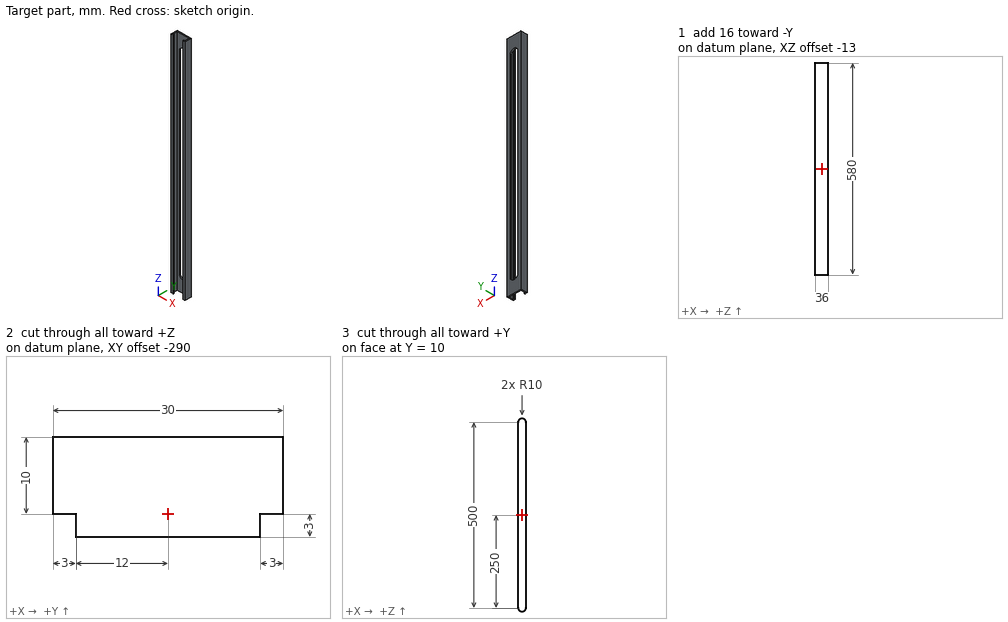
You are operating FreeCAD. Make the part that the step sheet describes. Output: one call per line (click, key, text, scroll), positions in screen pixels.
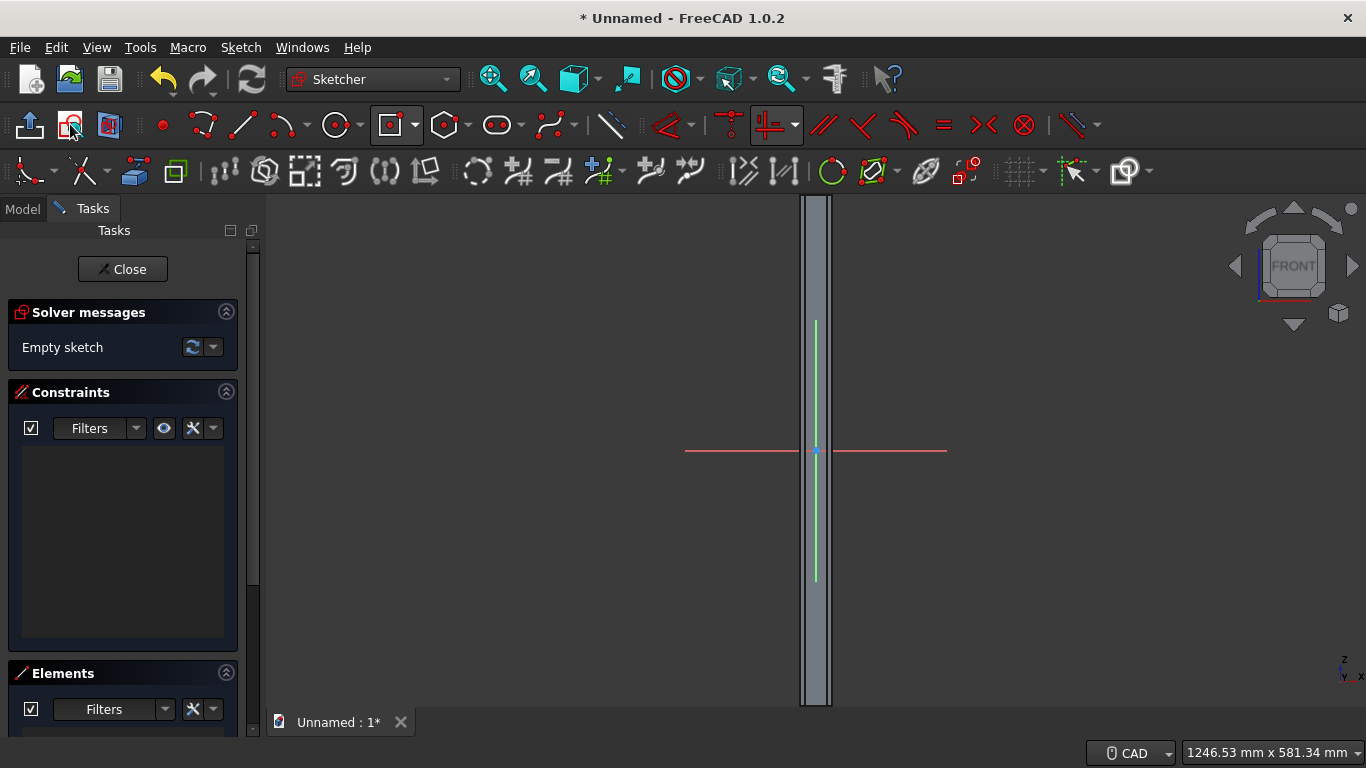
click(110, 126)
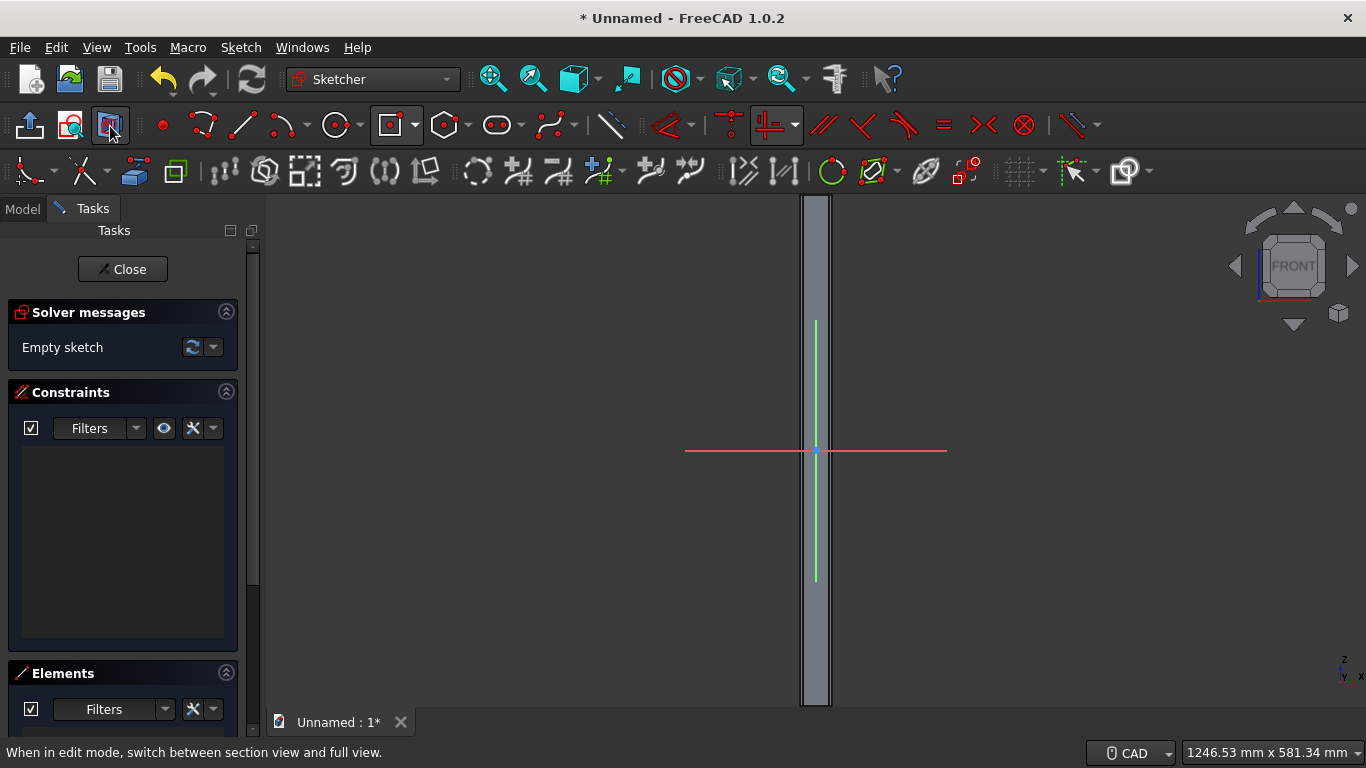
scroll(608, 450, down, 2)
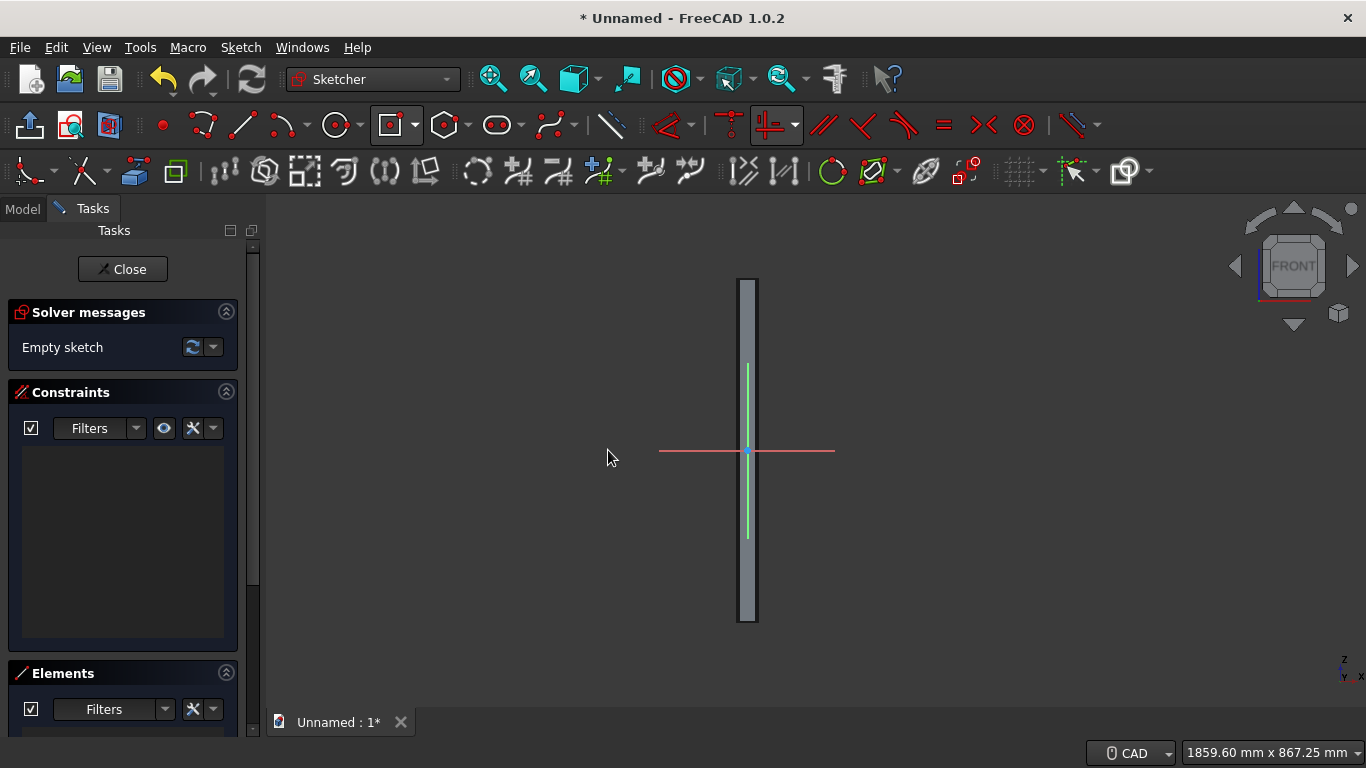
click(498, 126)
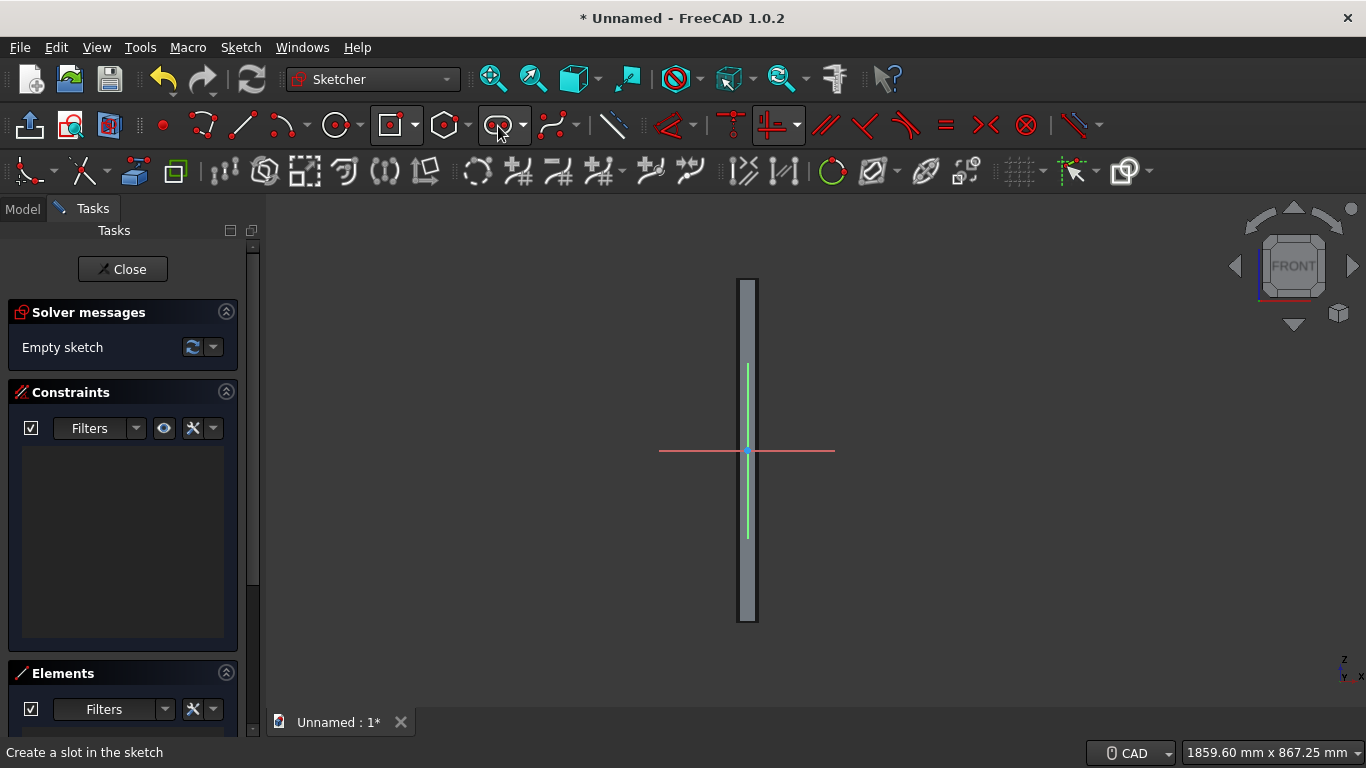
scroll(748, 598, up, 7)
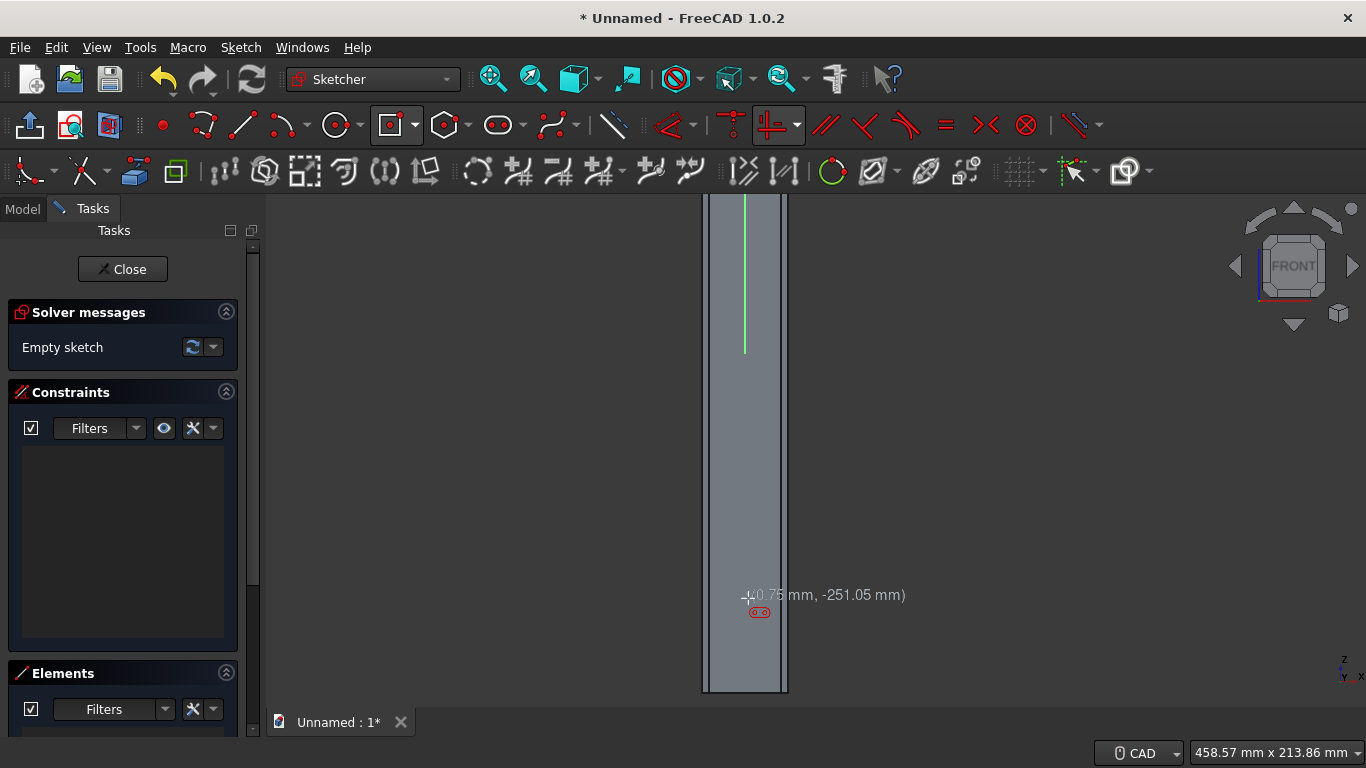
scroll(748, 599, down, 7)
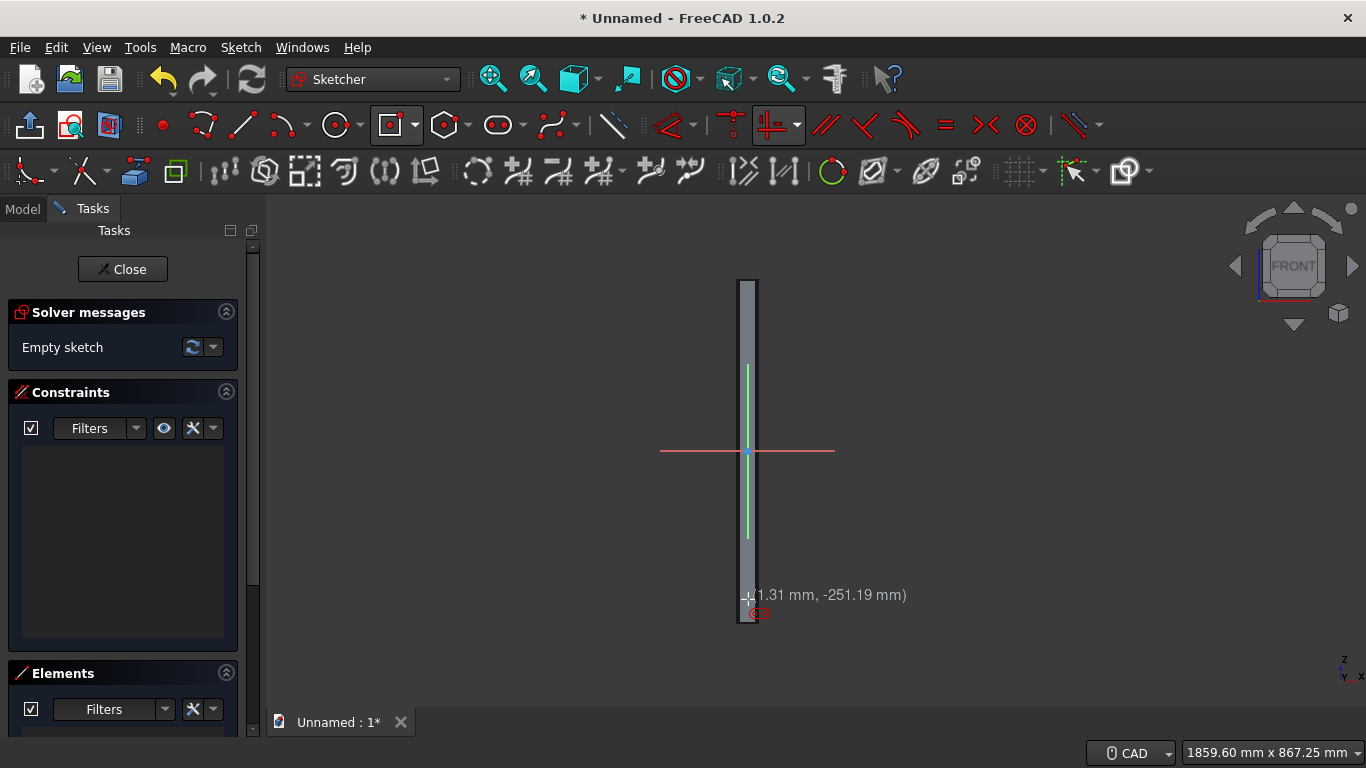
click(748, 599)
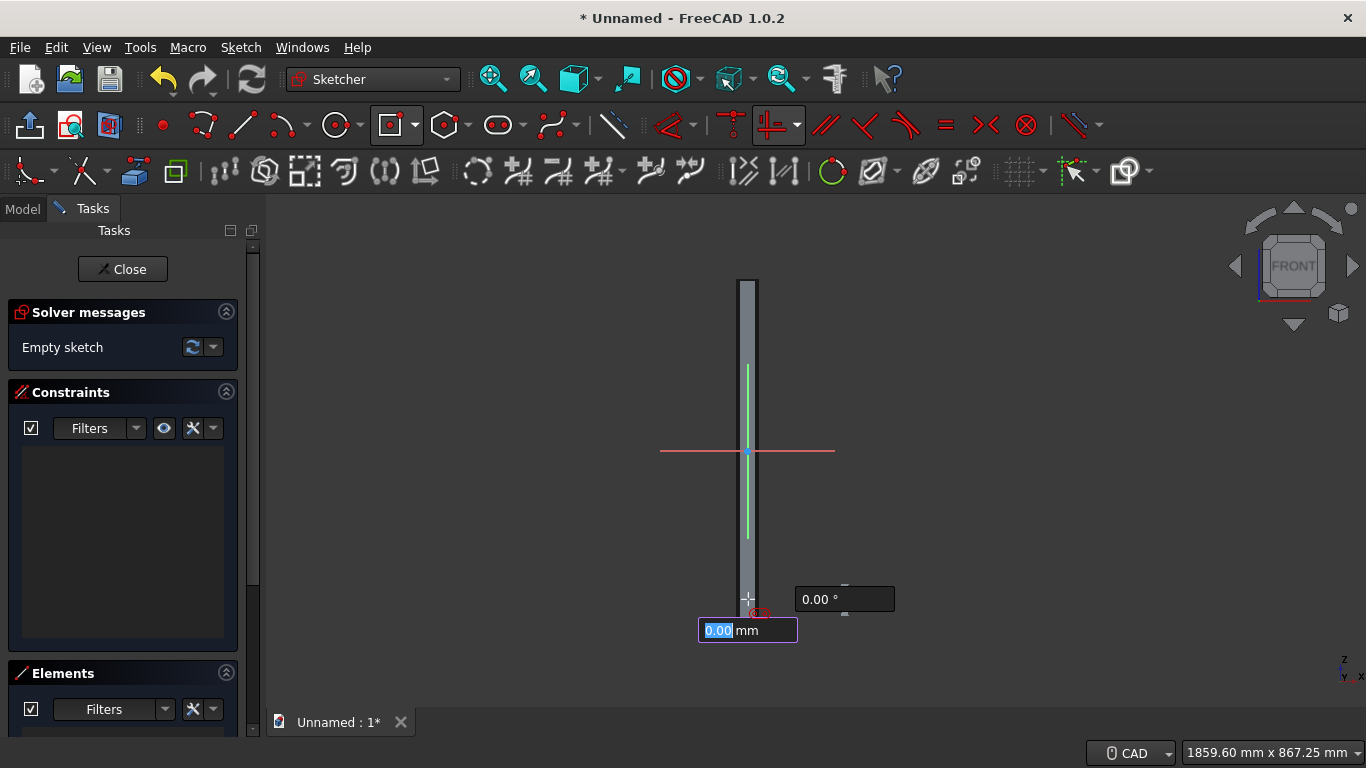
click(757, 303)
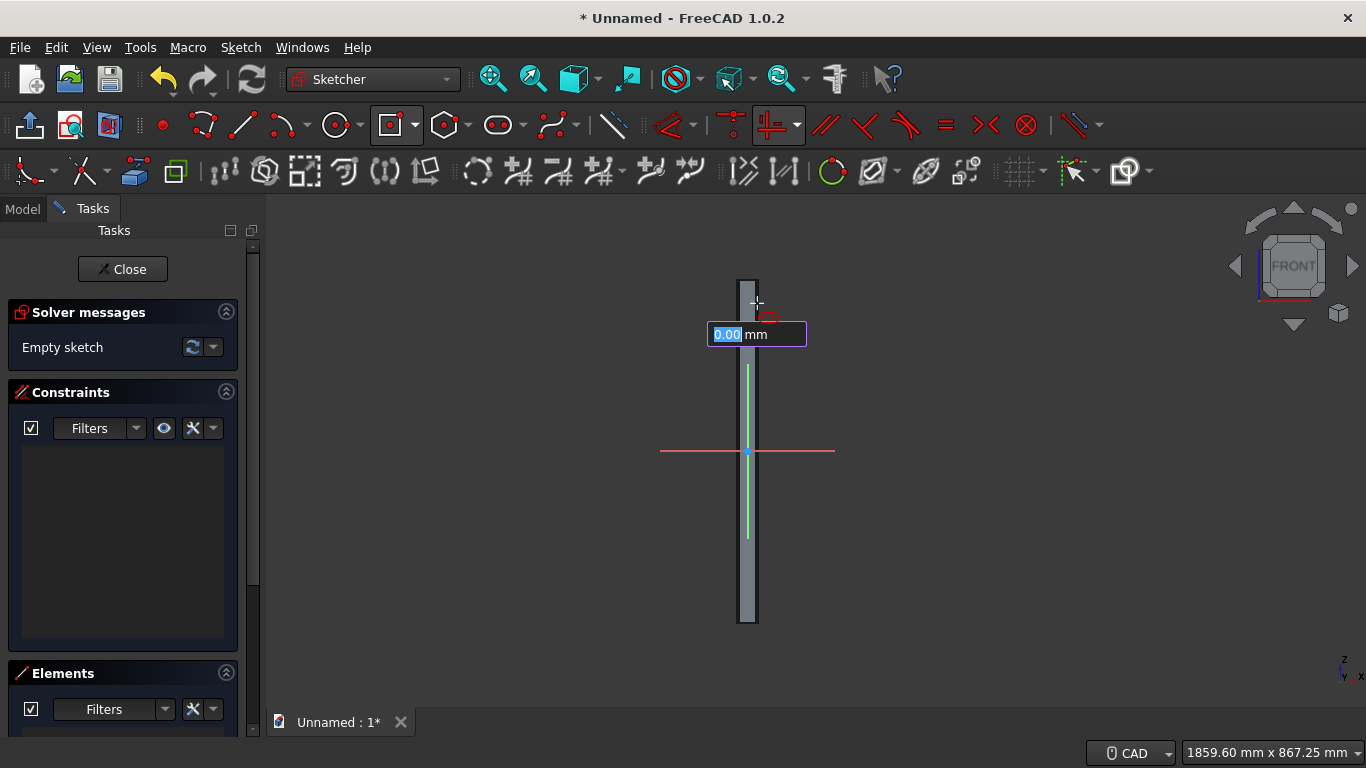
scroll(753, 496, up, 5)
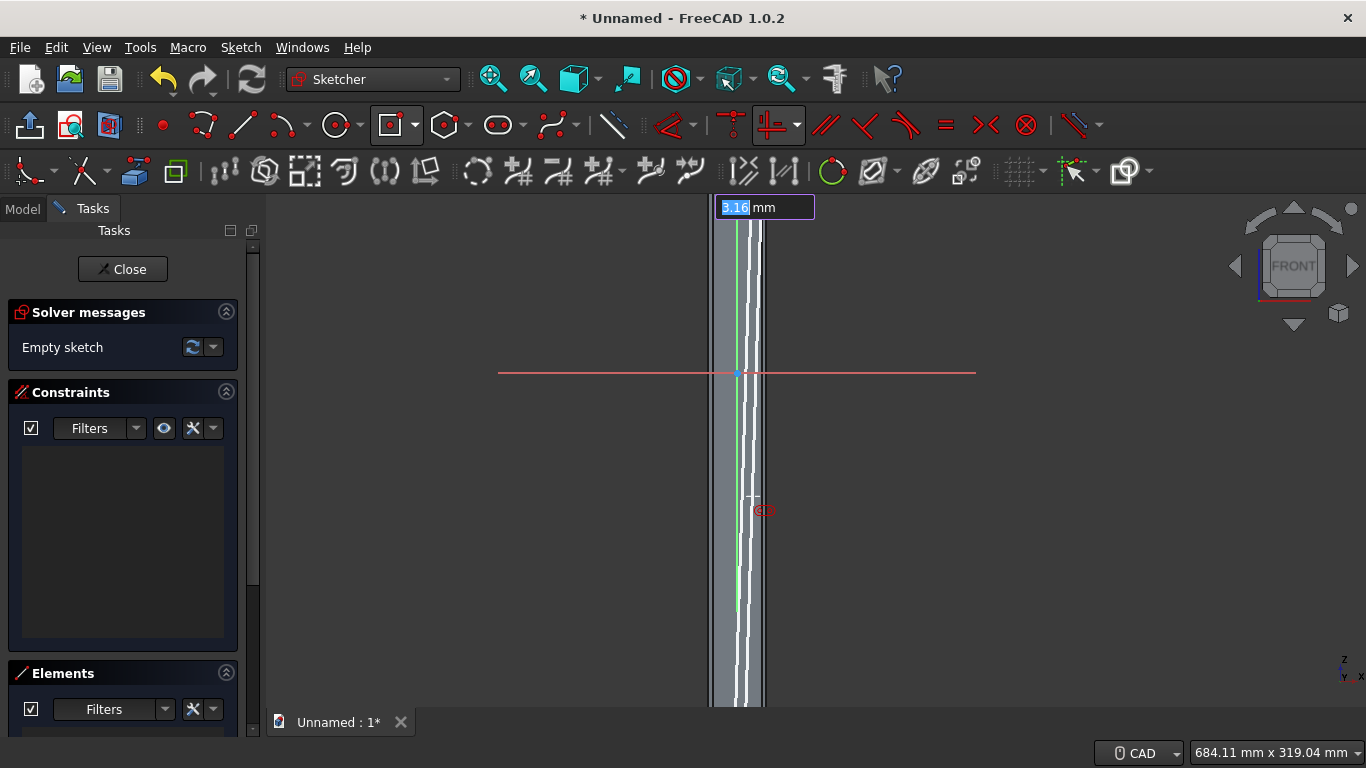
click(754, 494)
key(Escape)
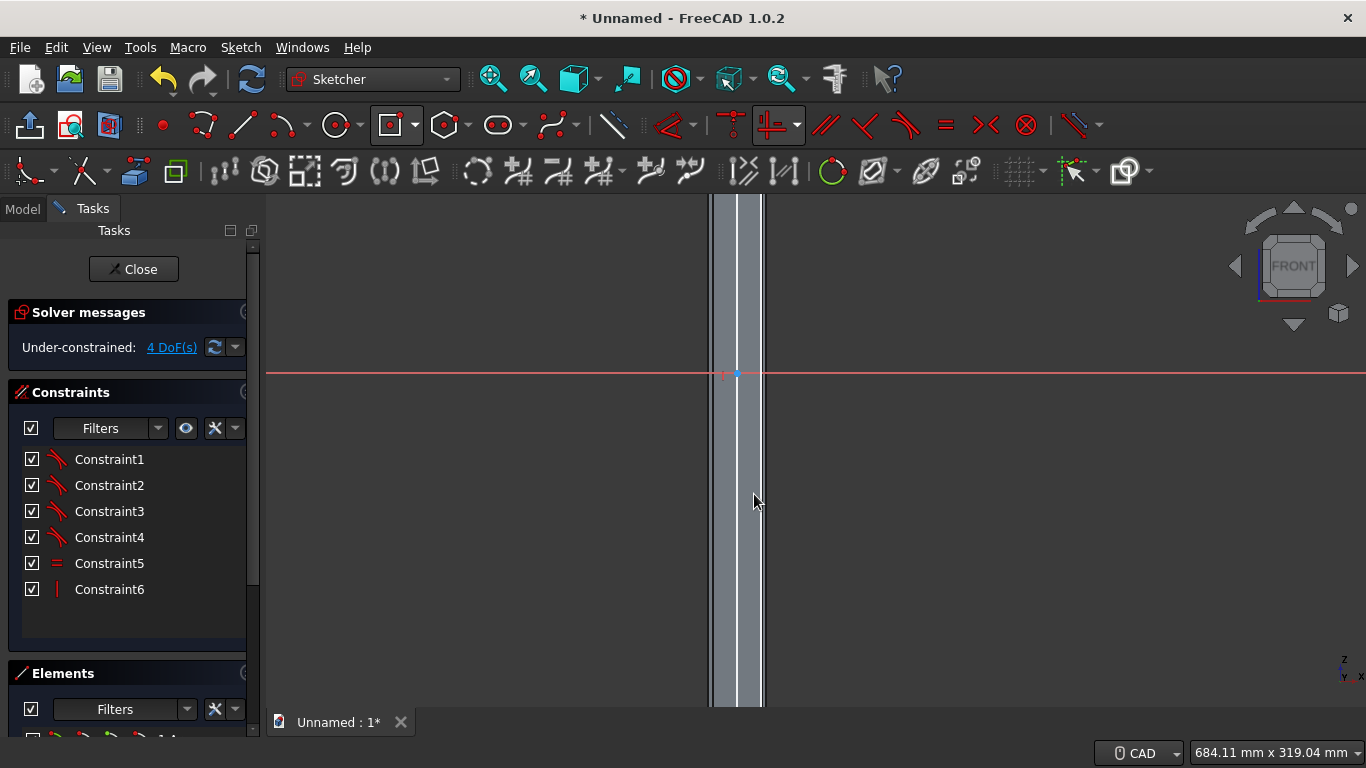
scroll(753, 495, down, 5)